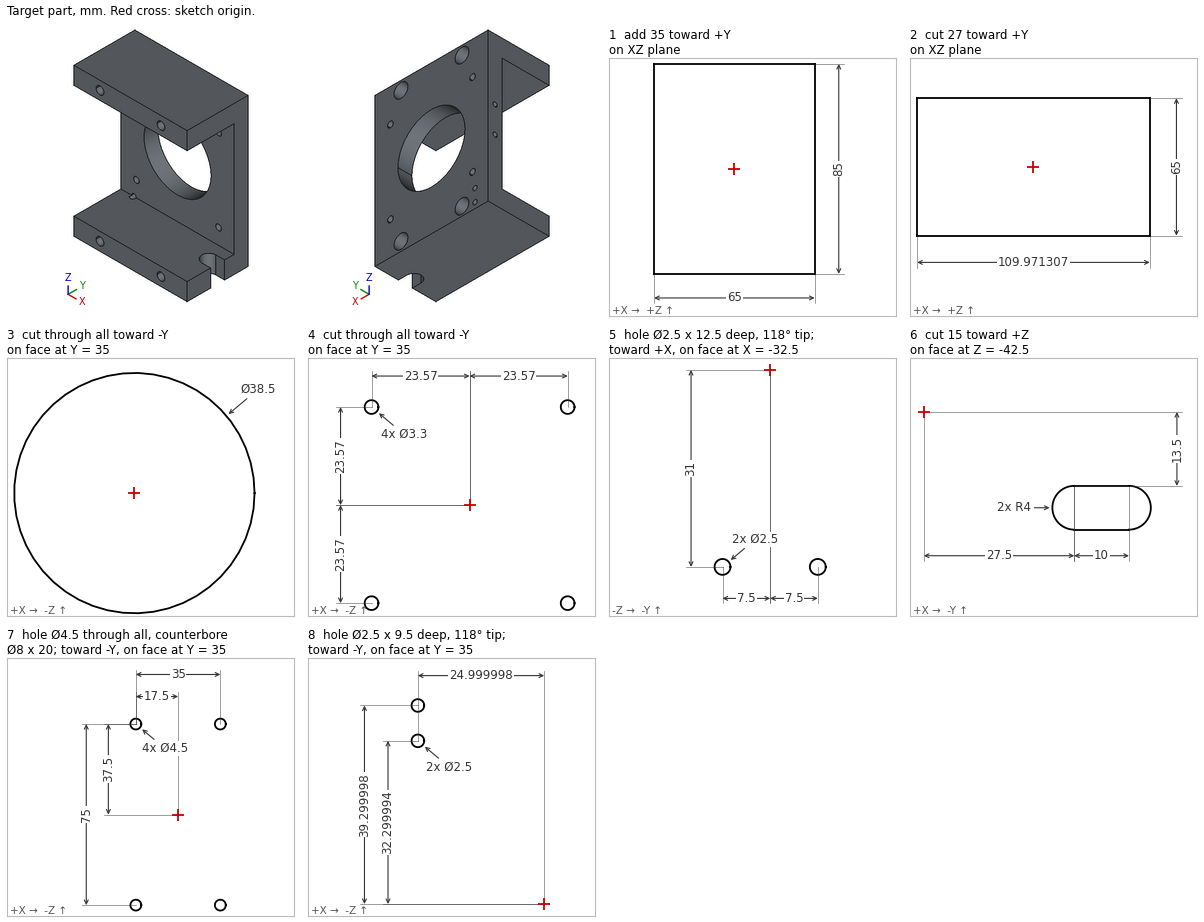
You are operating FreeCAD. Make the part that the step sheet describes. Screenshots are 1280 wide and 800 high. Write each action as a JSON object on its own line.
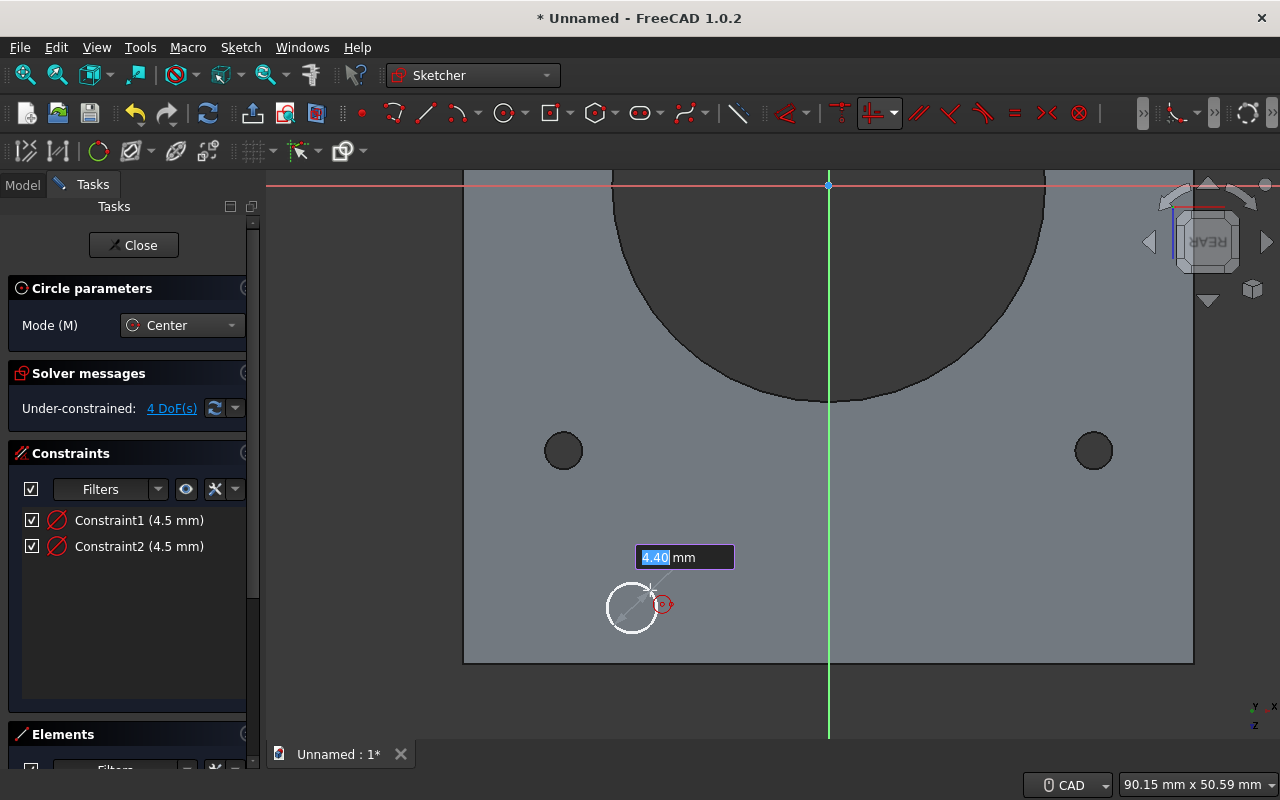
{"action": "type", "text": "4.5"}
{"action": "key", "text": "Return"}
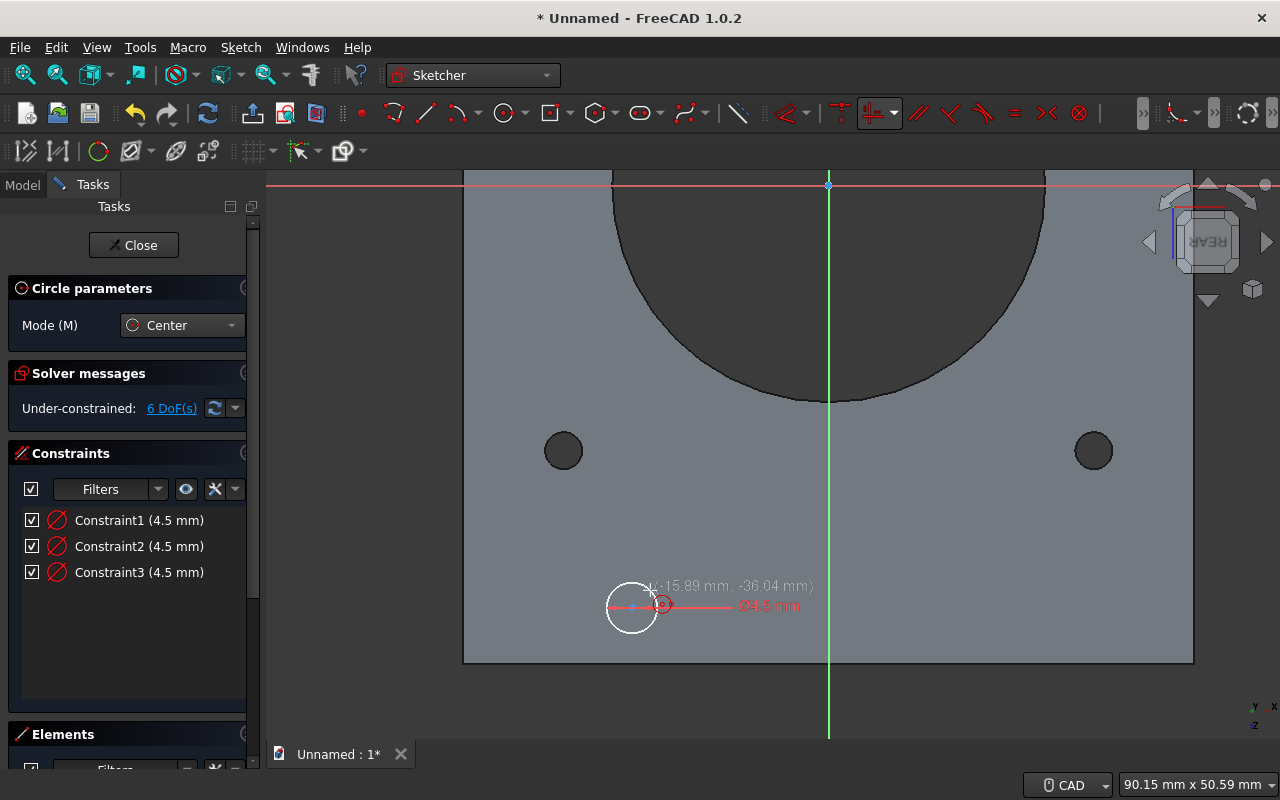
{"action": "left_click", "coordinate": [1026, 607]}
{"action": "mouse_move", "coordinate": [1043, 590]}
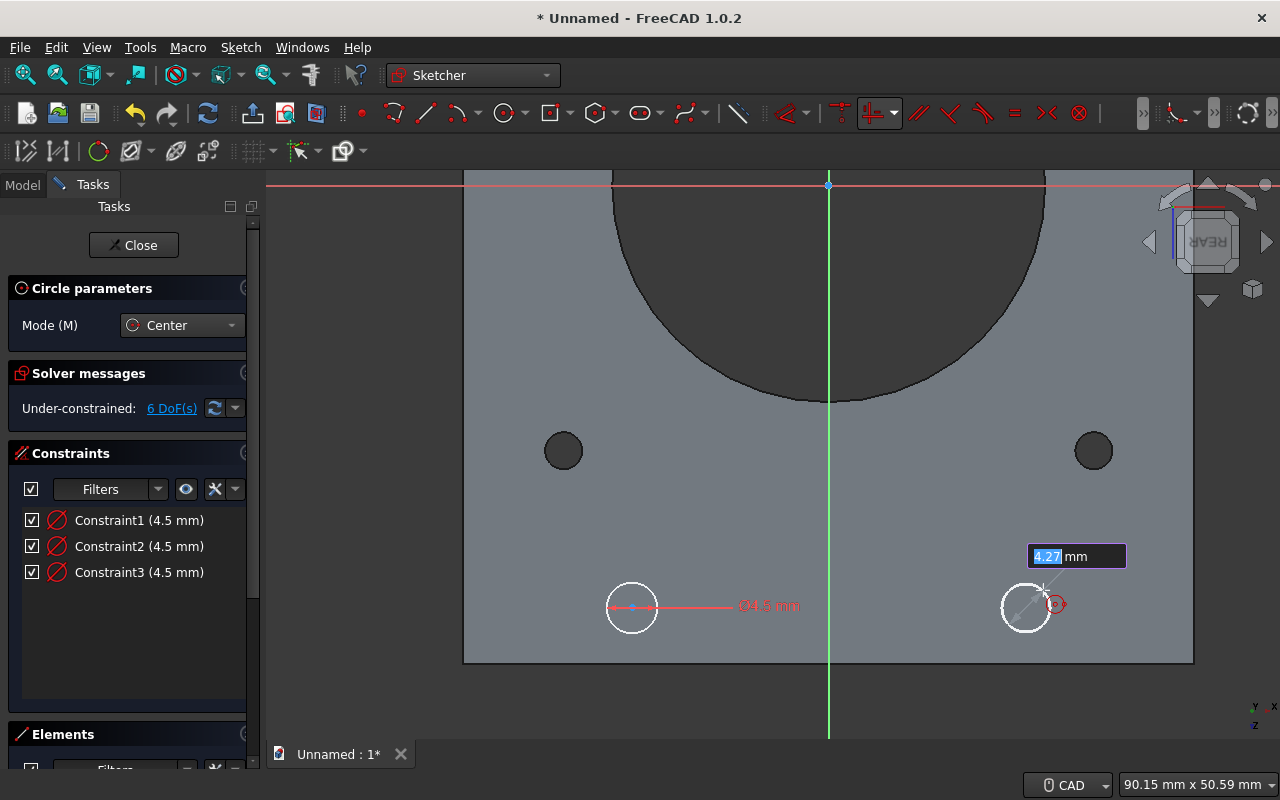
{"action": "type", "text": "4.5"}
{"action": "key", "text": "Return"}
{"action": "key", "text": "Escape"}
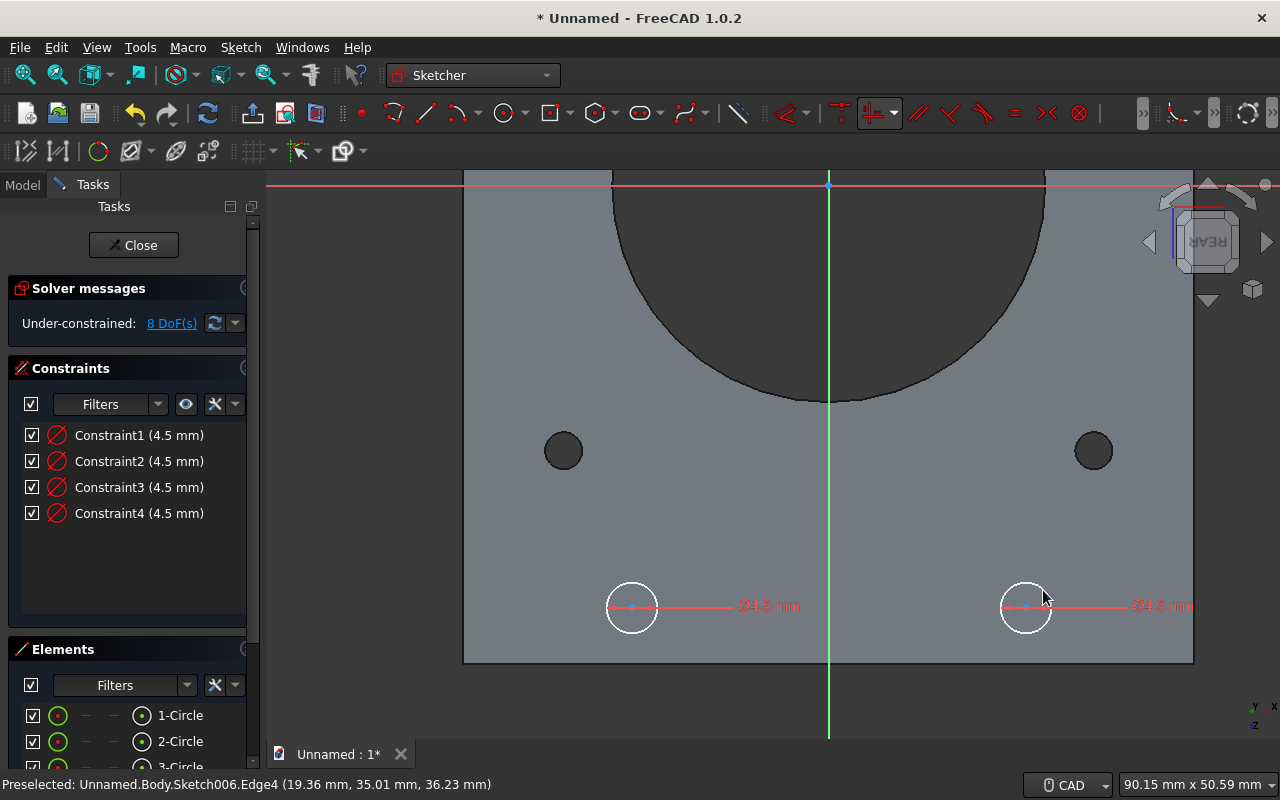
{"action": "scroll", "coordinate": [632, 611], "scroll_direction": "down", "scroll_amount": 5}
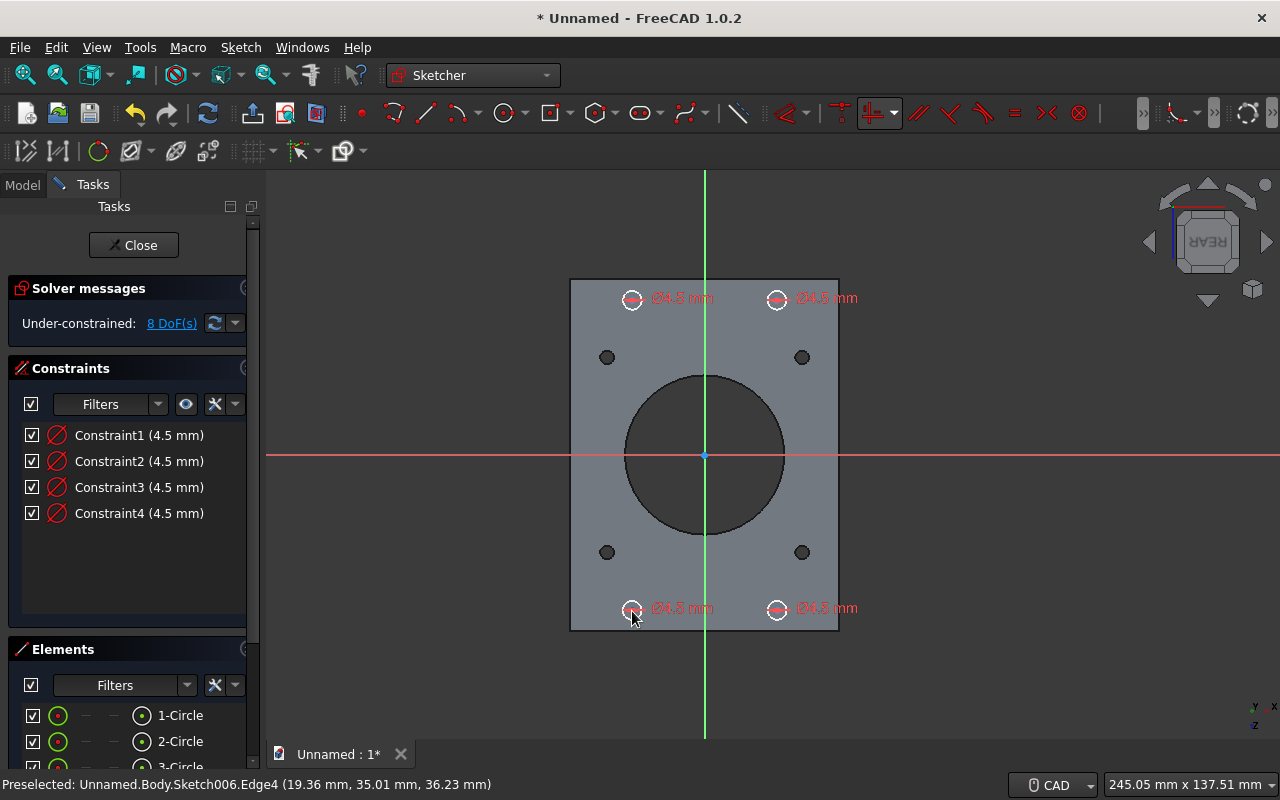
{"action": "left_click", "coordinate": [632, 300]}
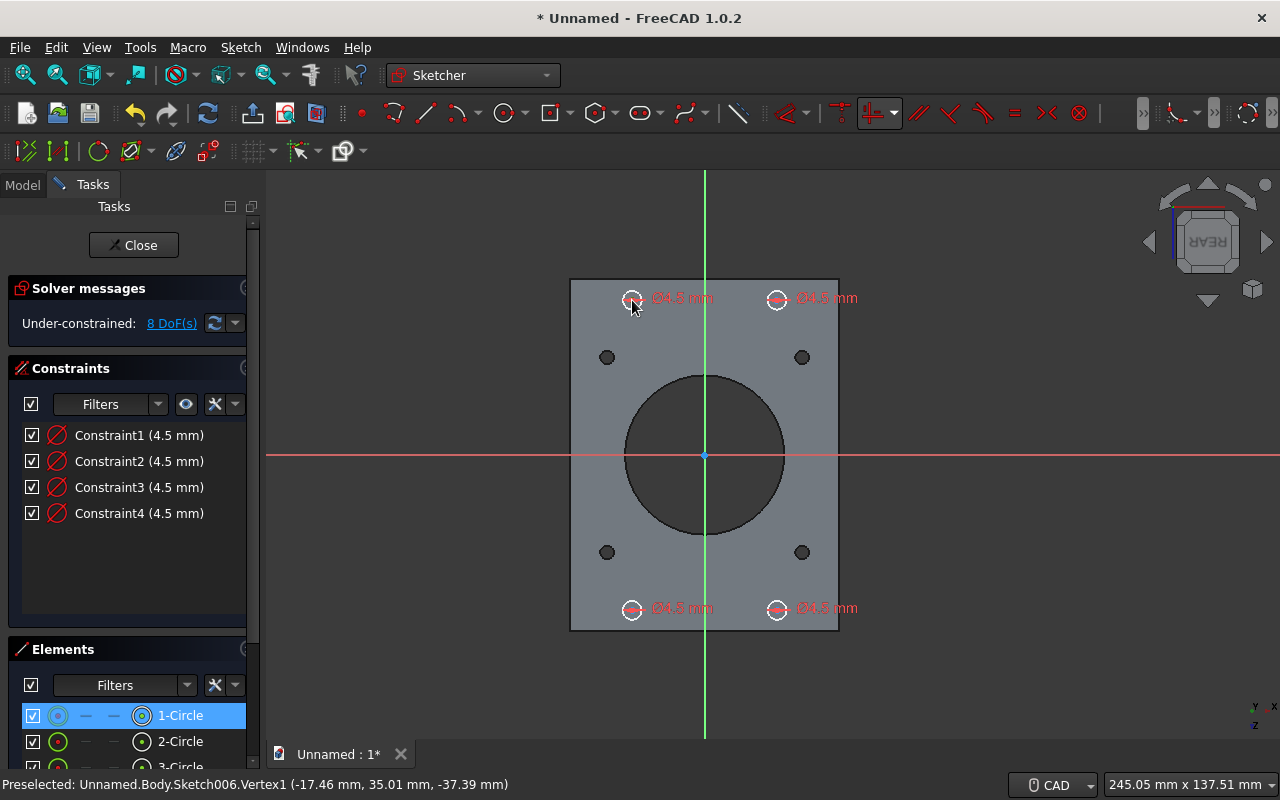
{"action": "left_click", "coordinate": [777, 300]}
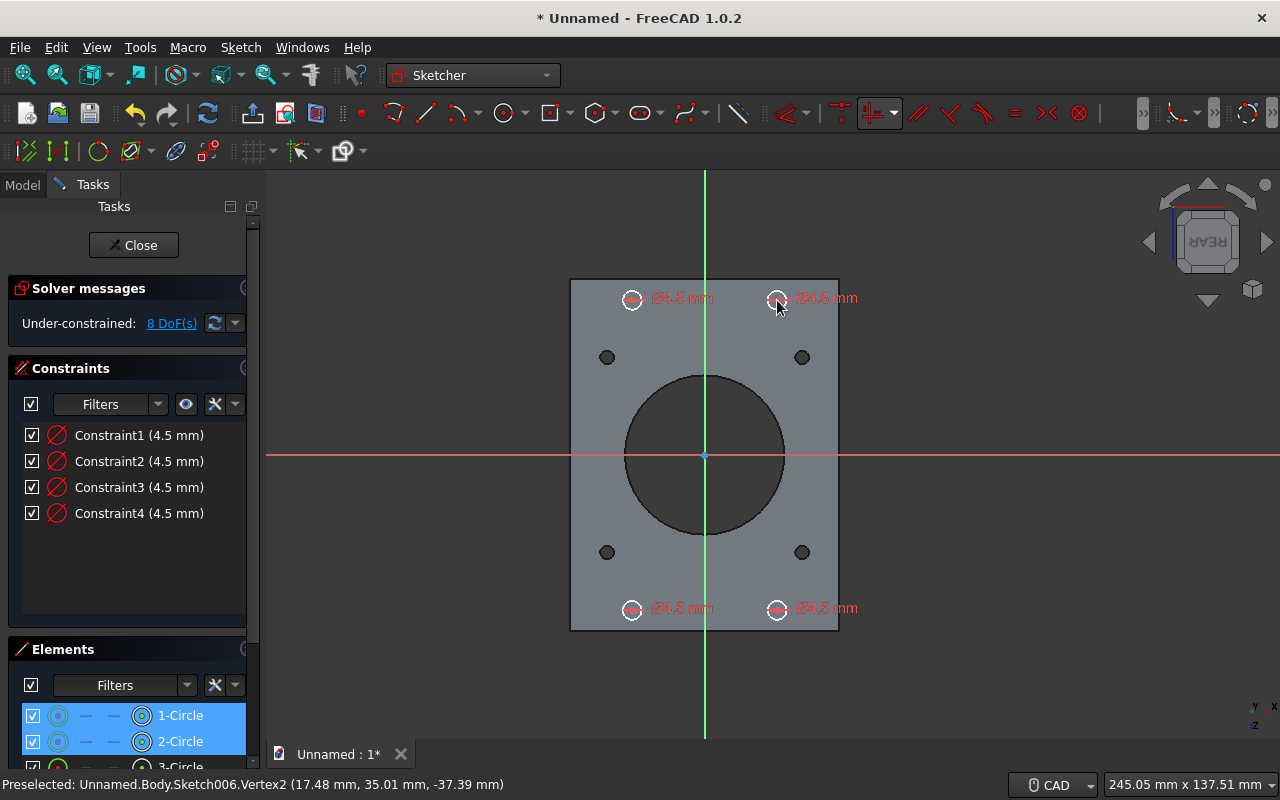
{"action": "key", "text": "h"}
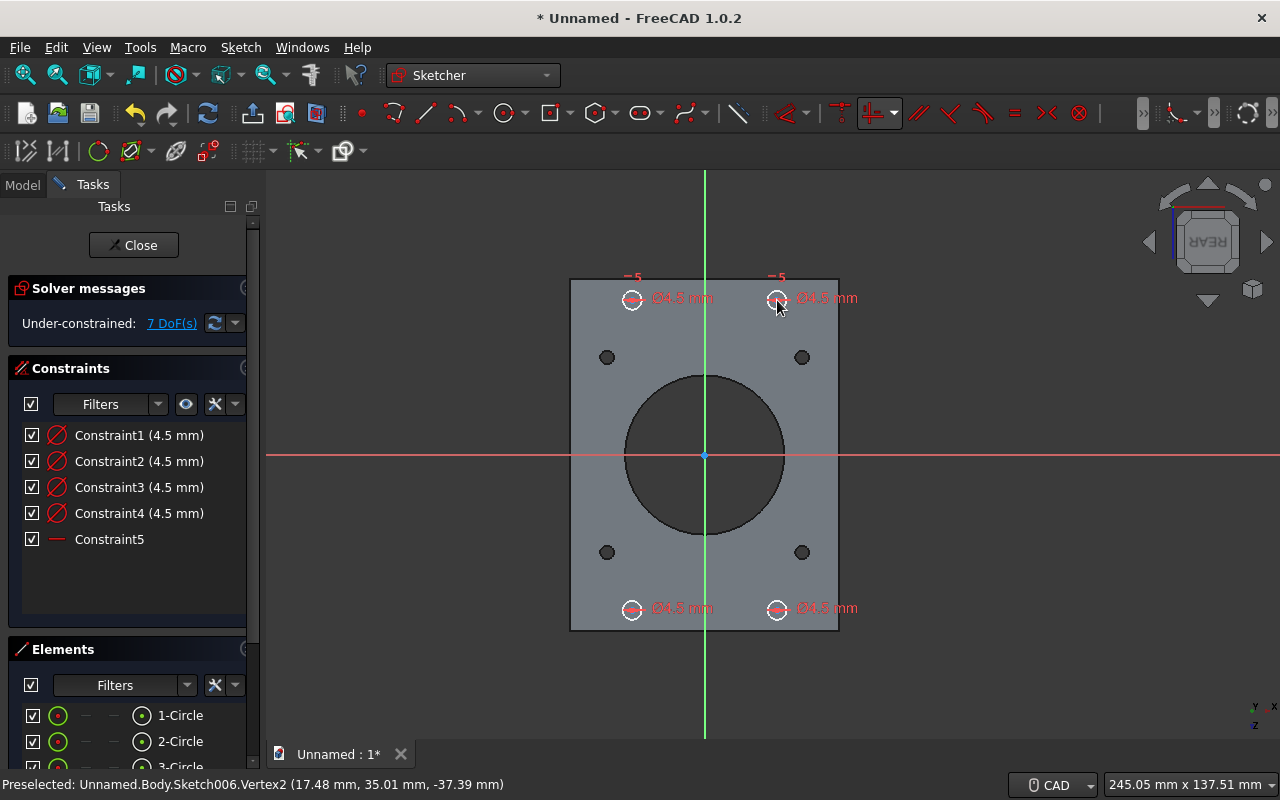
{"action": "left_click", "coordinate": [632, 300]}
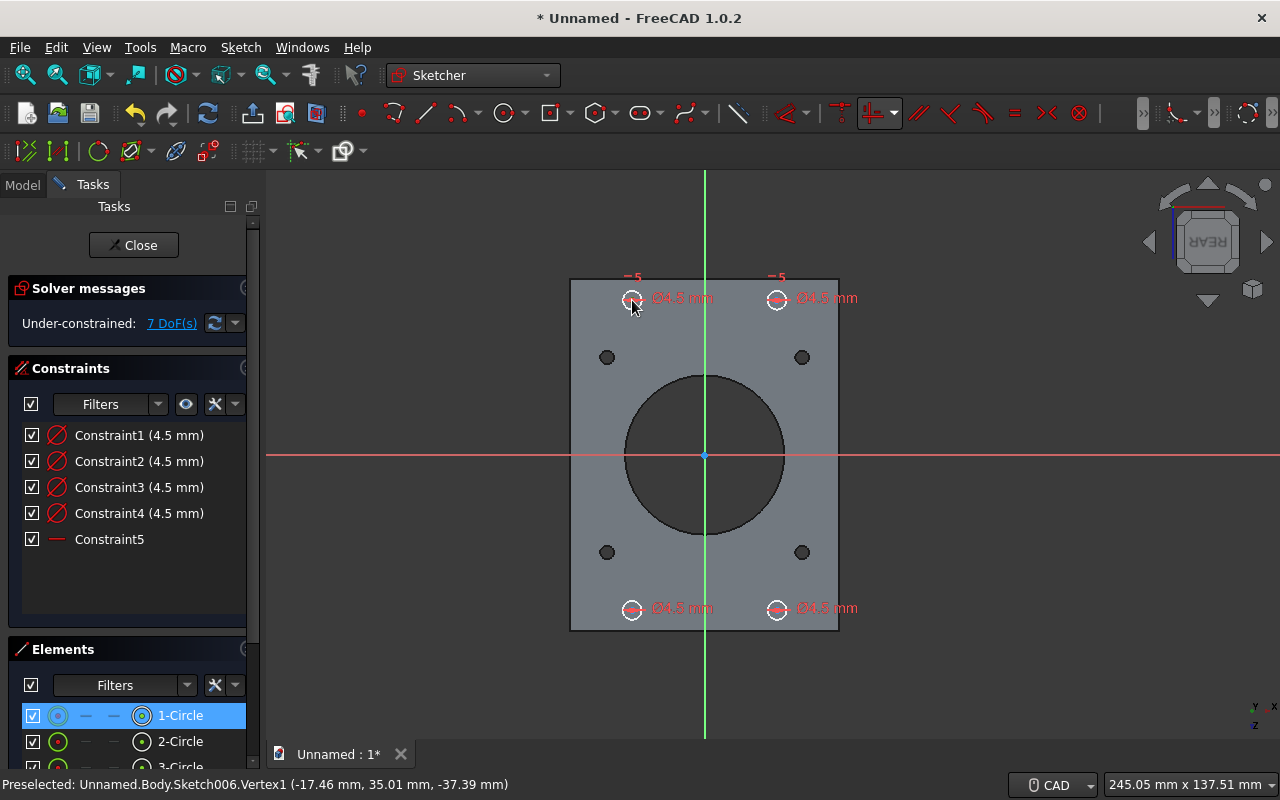
{"action": "left_click", "coordinate": [632, 610]}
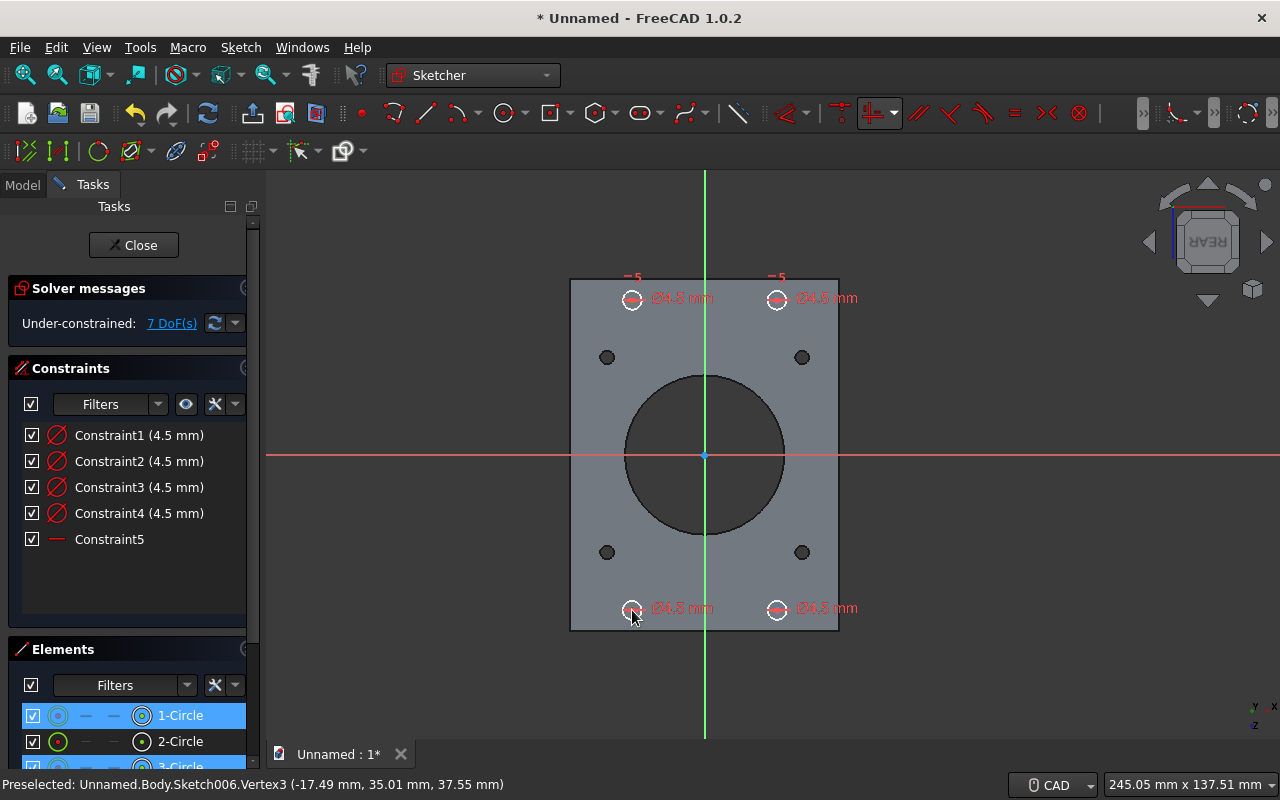
{"action": "left_click", "coordinate": [896, 114]}